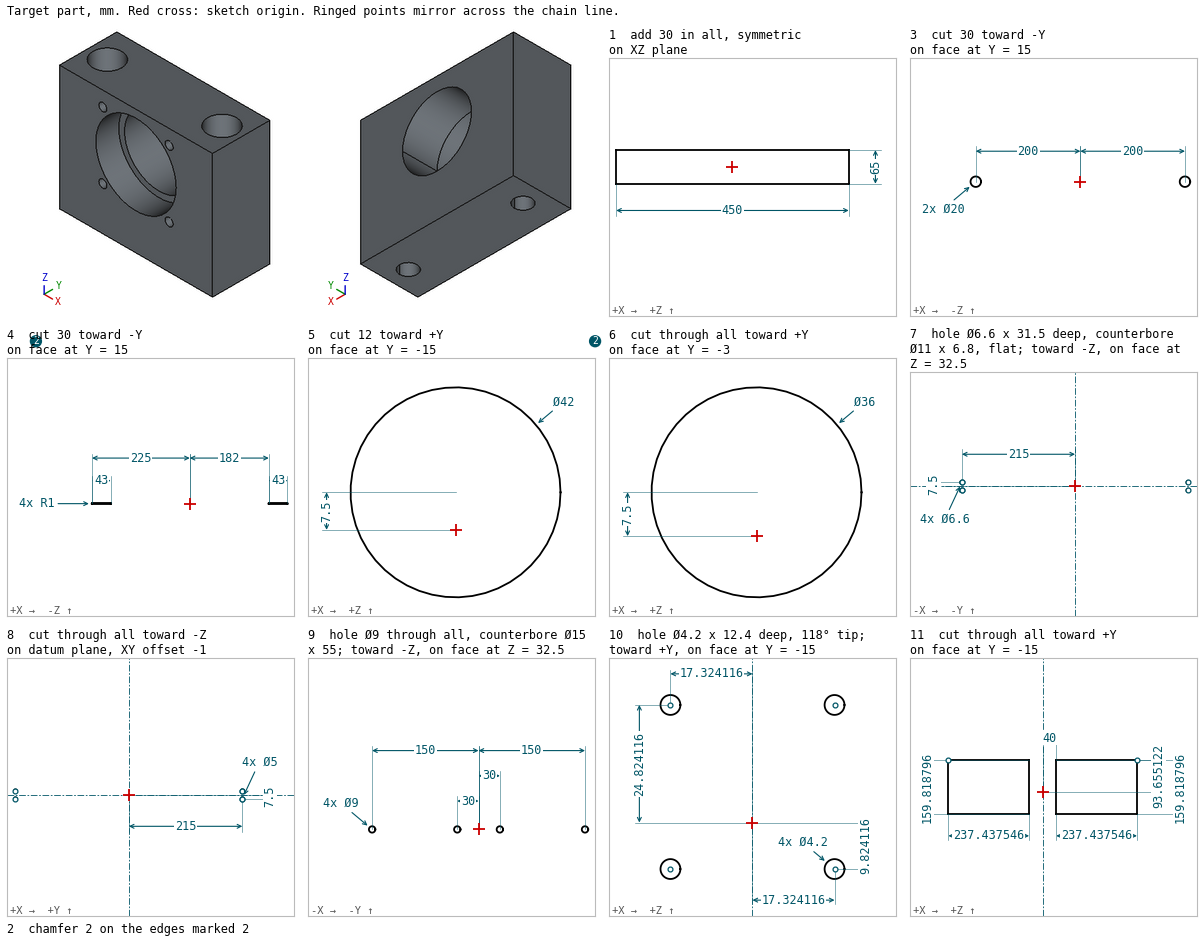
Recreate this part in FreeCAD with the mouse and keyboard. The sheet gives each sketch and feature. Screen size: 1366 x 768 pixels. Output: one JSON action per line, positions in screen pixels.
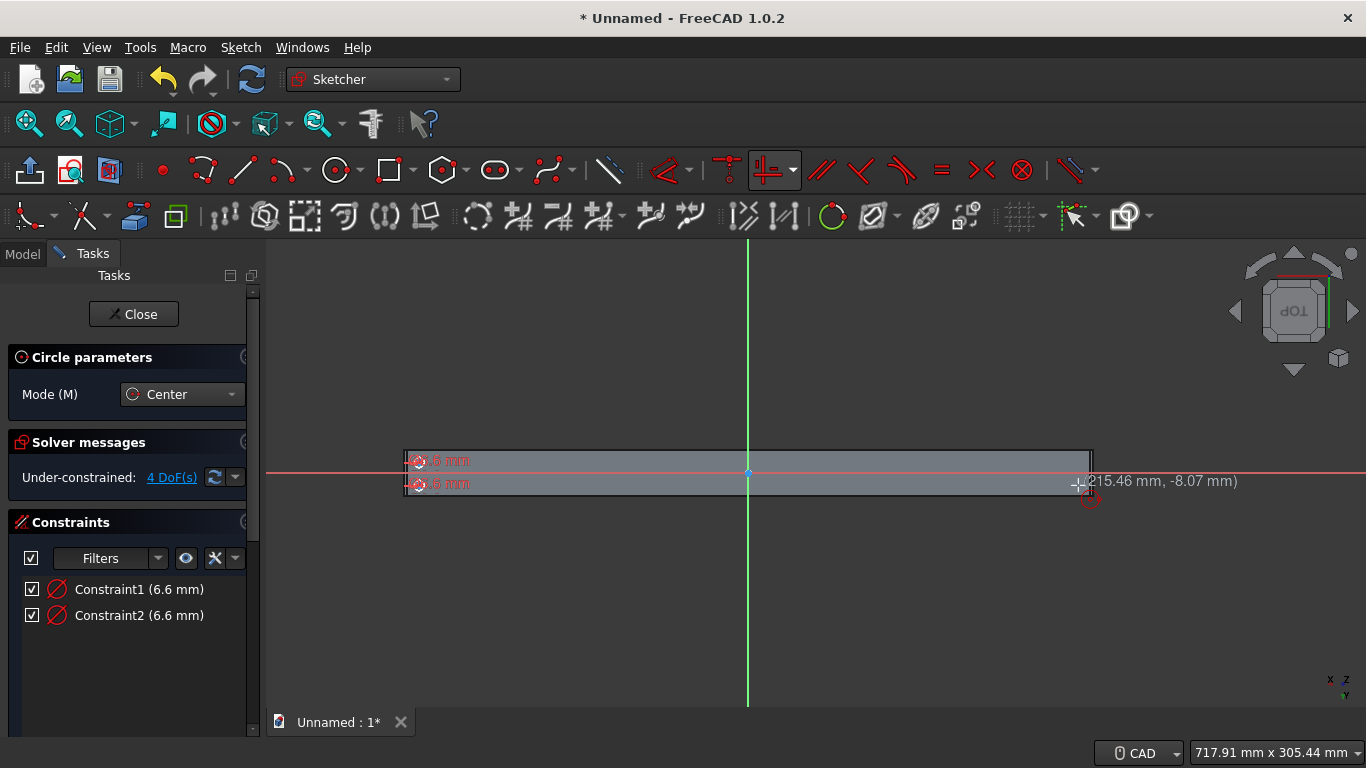
{"action": "scroll", "coordinate": [1078, 485], "scroll_direction": "up", "scroll_amount": 2}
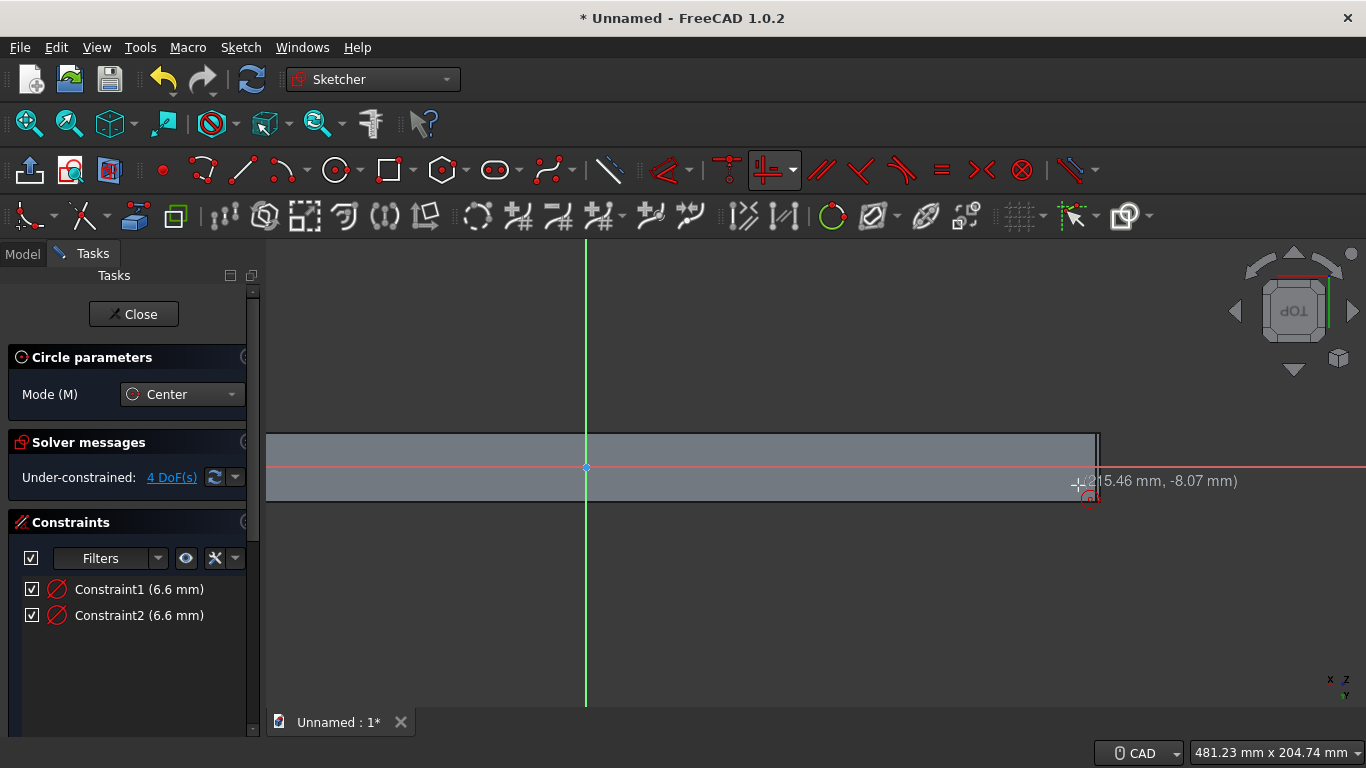
{"action": "left_click", "coordinate": [1077, 484]}
{"action": "mouse_move", "coordinate": [1083, 490]}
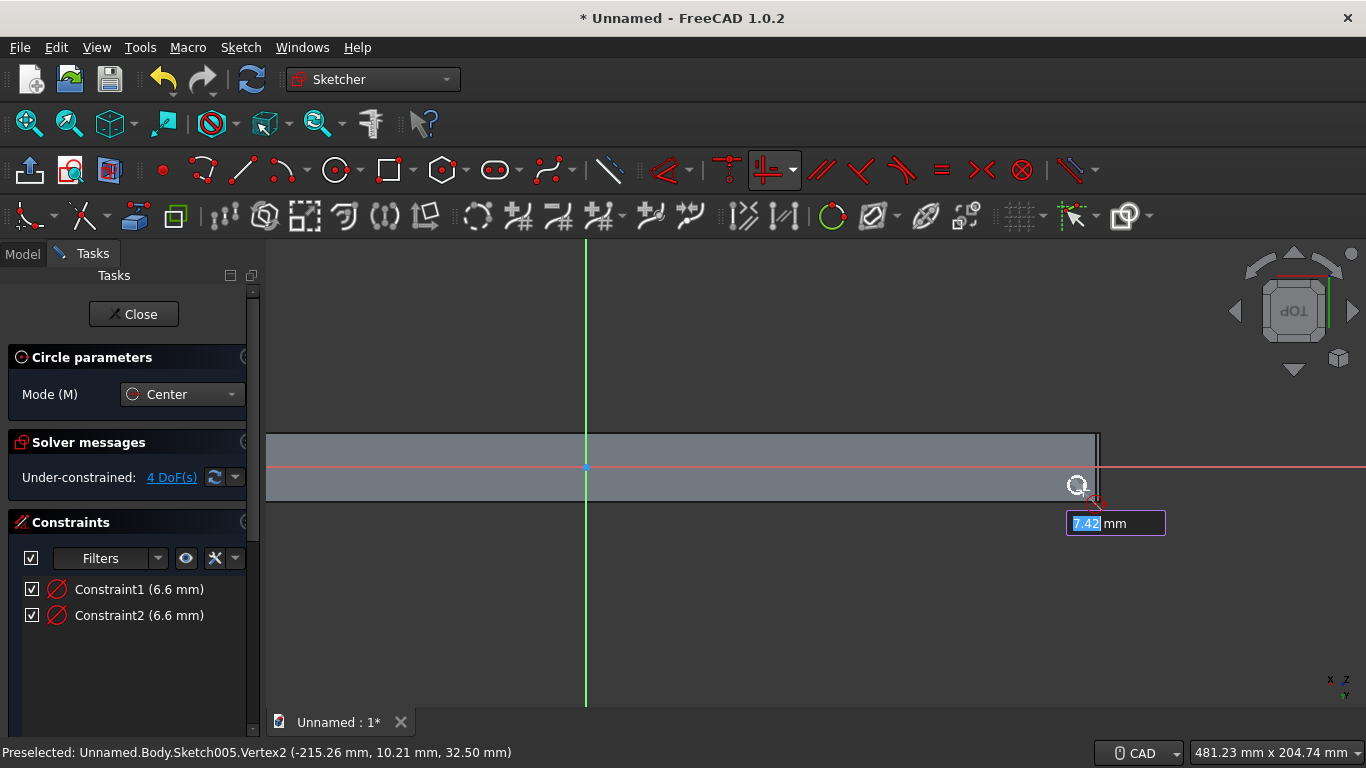
{"action": "type", "text": "6.6"}
{"action": "key", "text": "Return"}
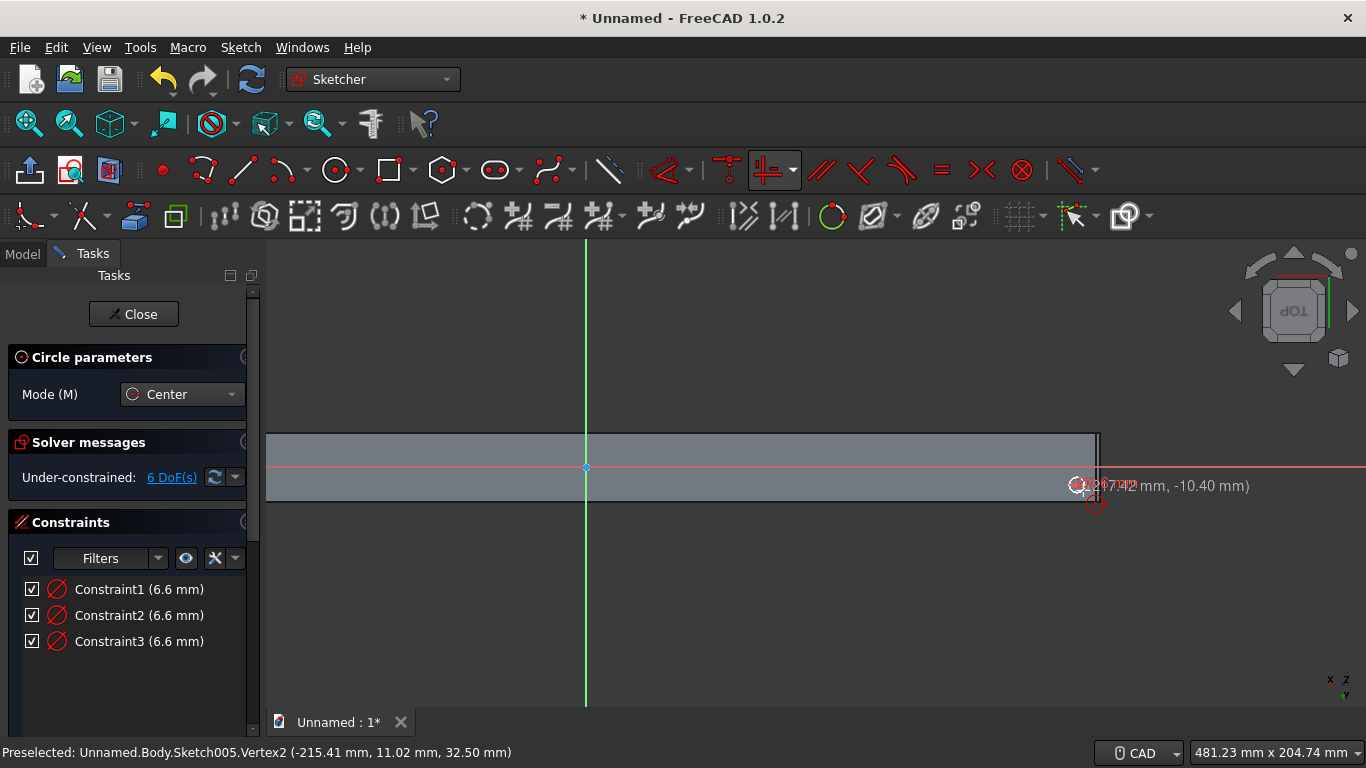
{"action": "scroll", "coordinate": [1077, 450], "scroll_direction": "up", "scroll_amount": 6}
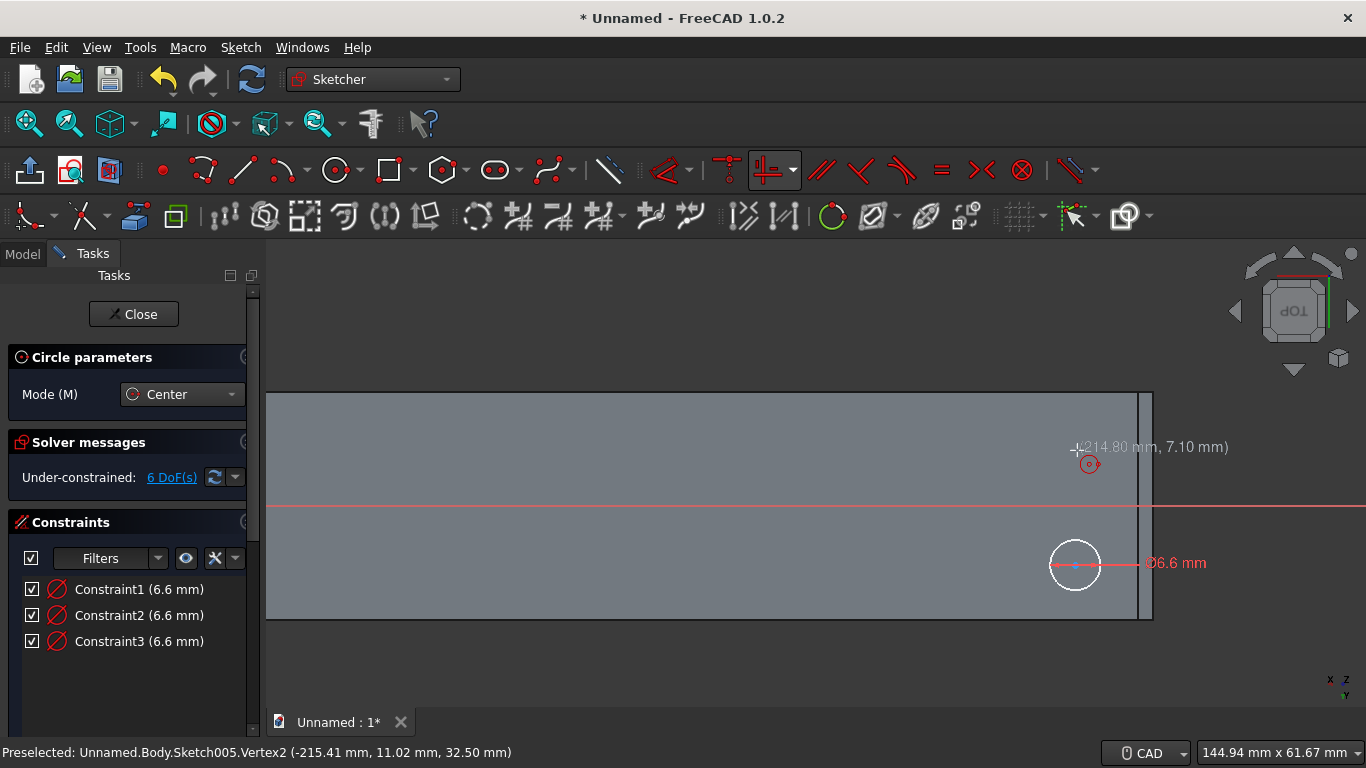
{"action": "scroll", "coordinate": [1077, 465], "scroll_direction": "down", "scroll_amount": 8}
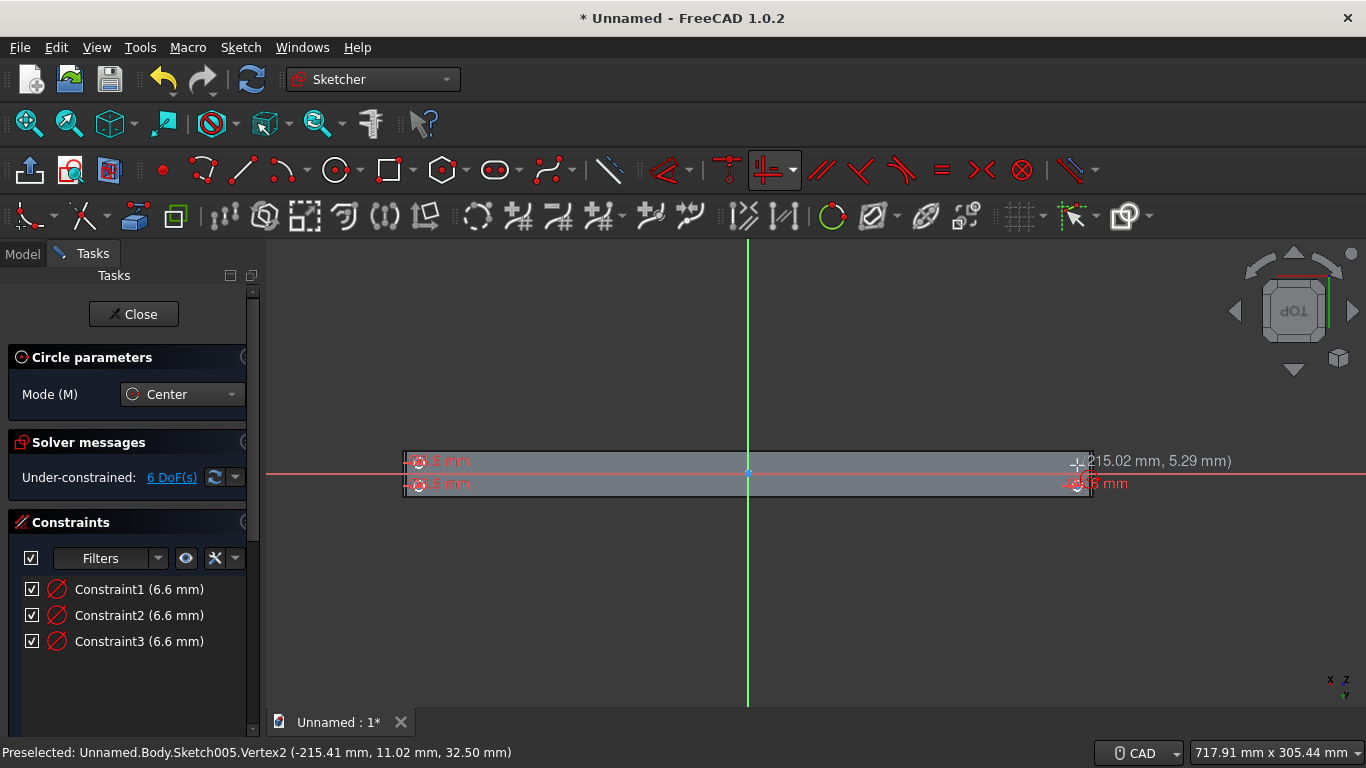
{"action": "scroll", "coordinate": [1078, 462], "scroll_direction": "up", "scroll_amount": 2}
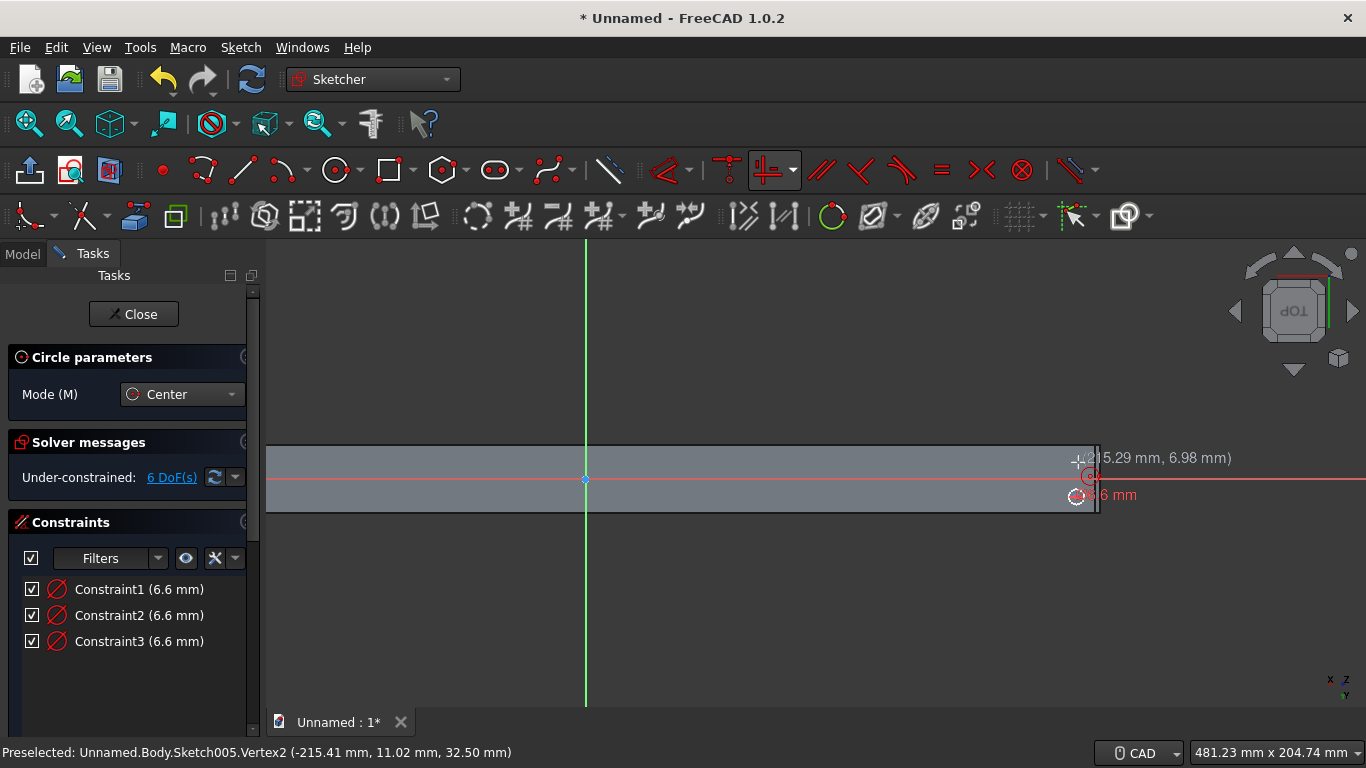
{"action": "left_click", "coordinate": [1077, 462]}
{"action": "mouse_move", "coordinate": [1082, 457]}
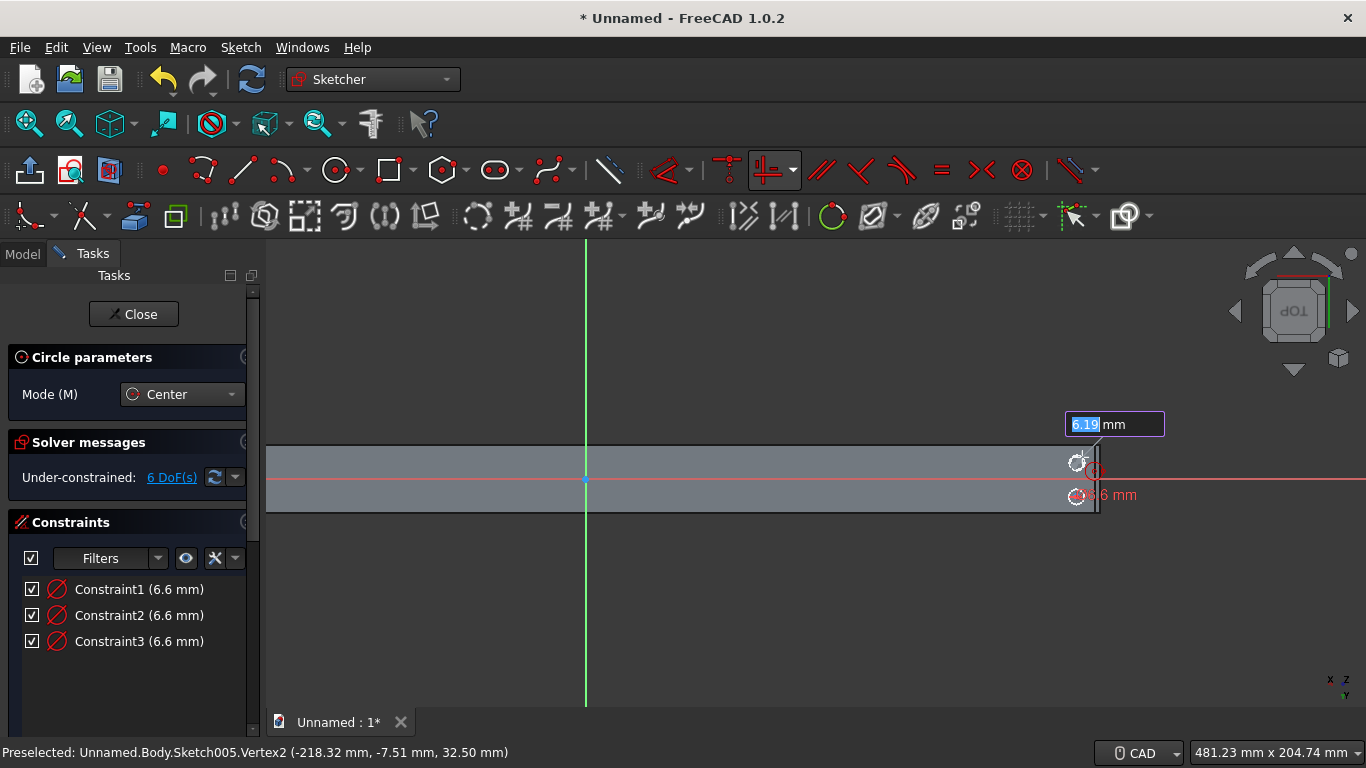
{"action": "type", "text": "6.6"}
{"action": "key", "text": "Return"}
{"action": "key", "text": "Escape"}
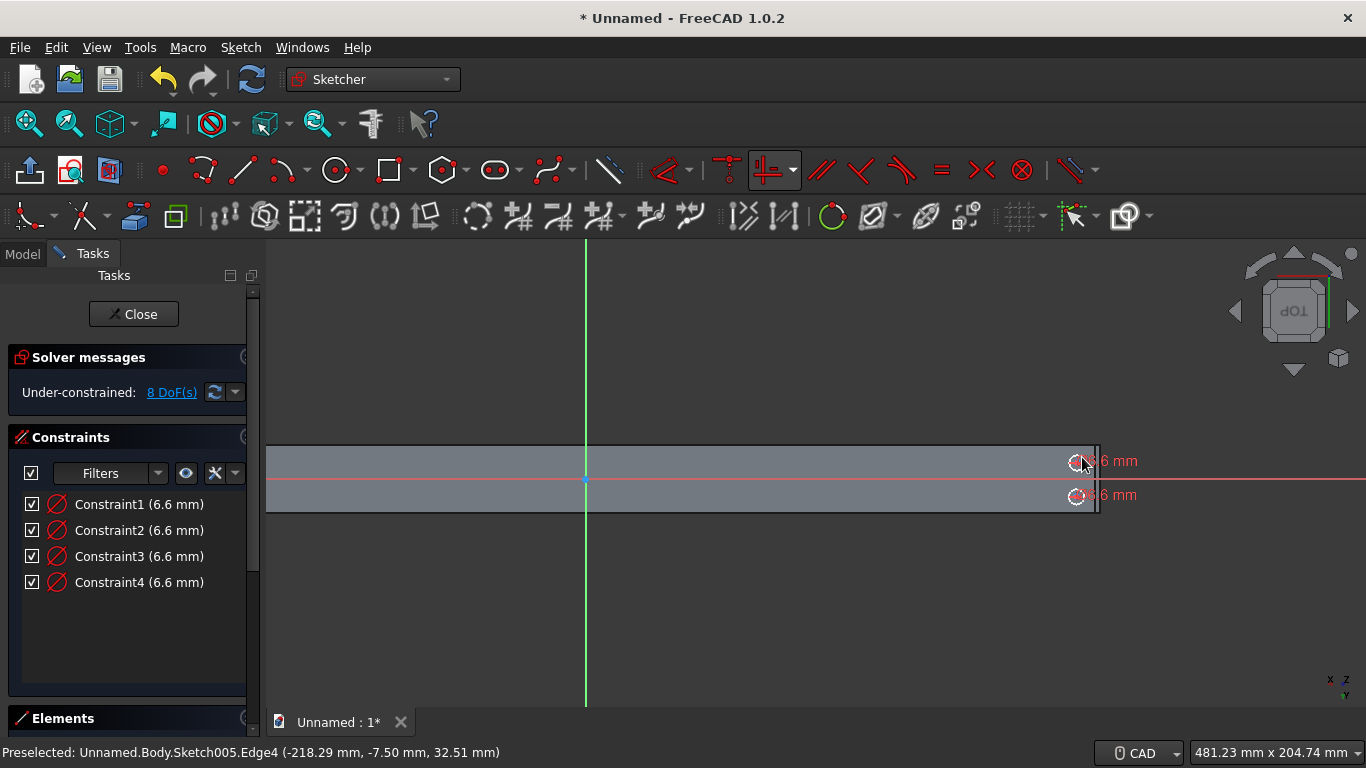
{"action": "scroll", "coordinate": [1077, 460], "scroll_direction": "down", "scroll_amount": 2}